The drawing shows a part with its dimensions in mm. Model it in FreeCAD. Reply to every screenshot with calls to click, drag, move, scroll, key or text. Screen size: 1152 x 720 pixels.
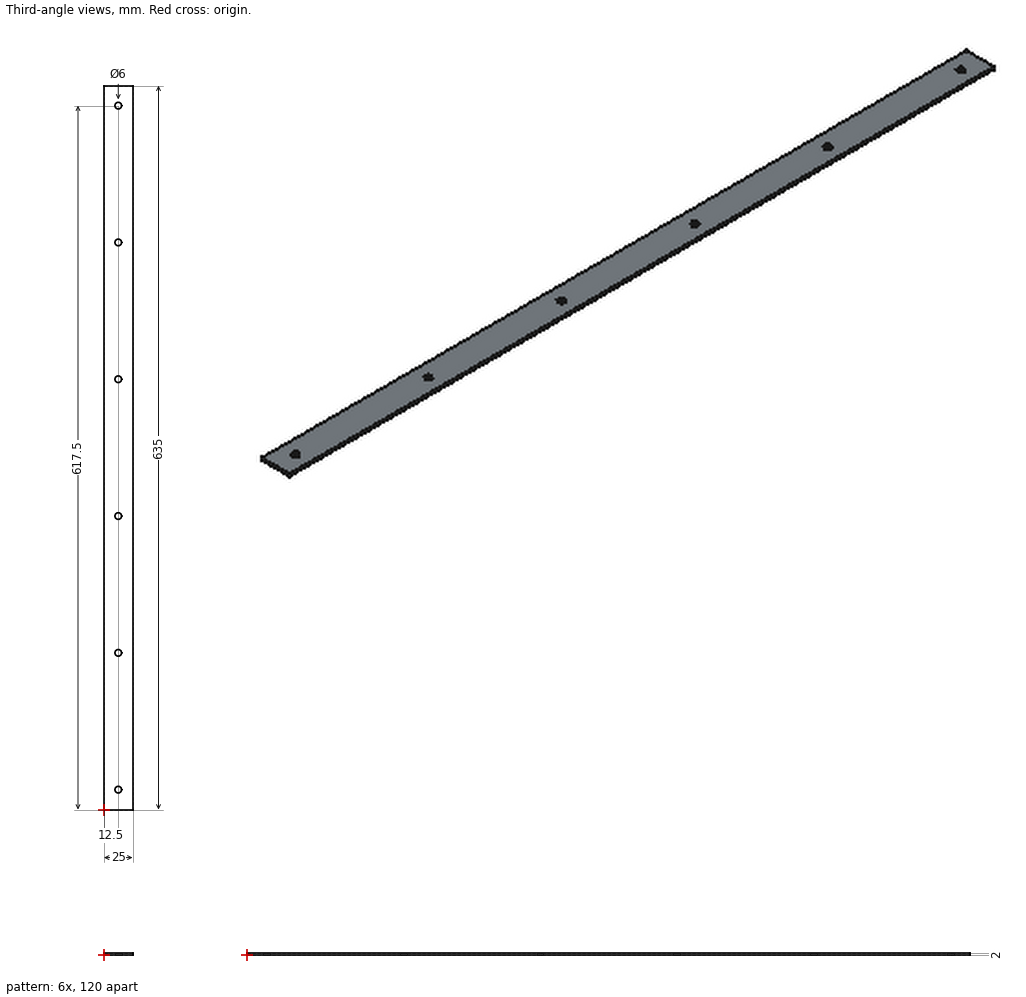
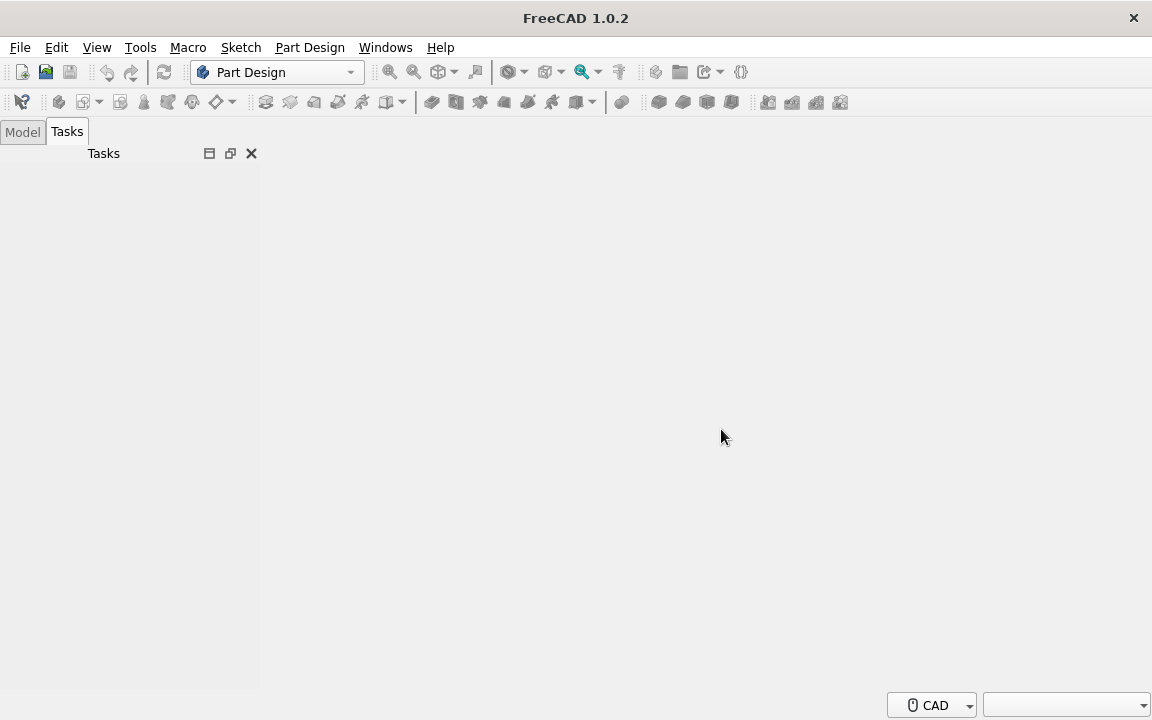
key(ctrl+n)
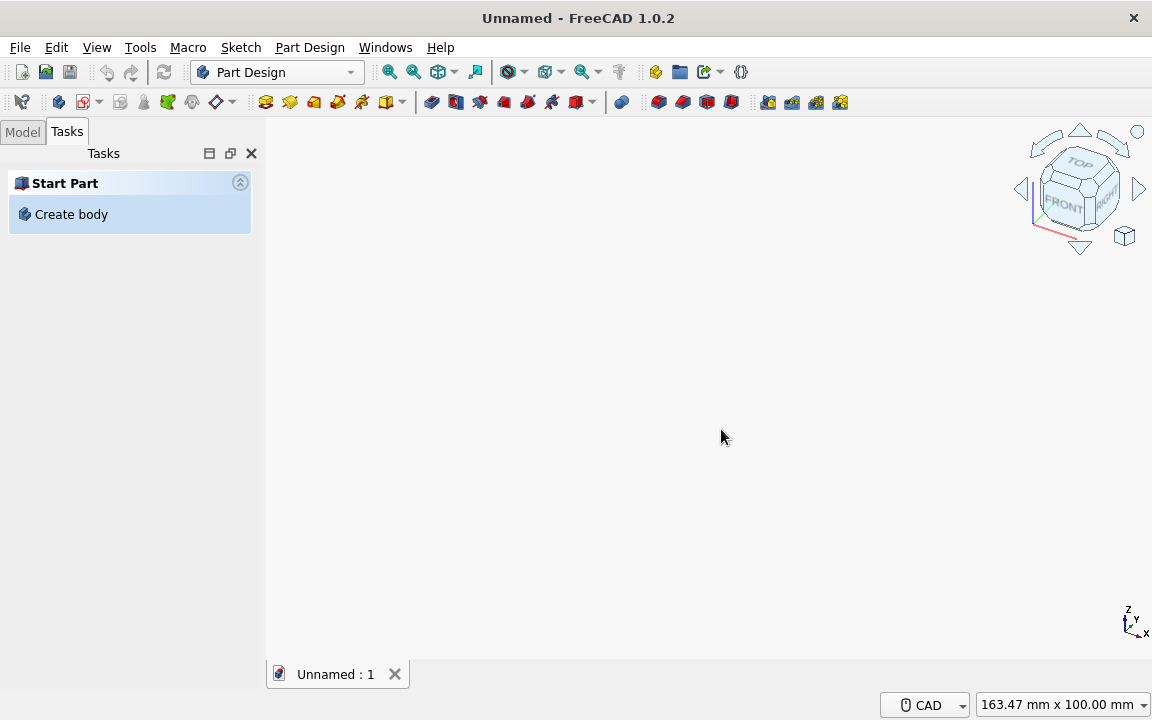
click(84, 102)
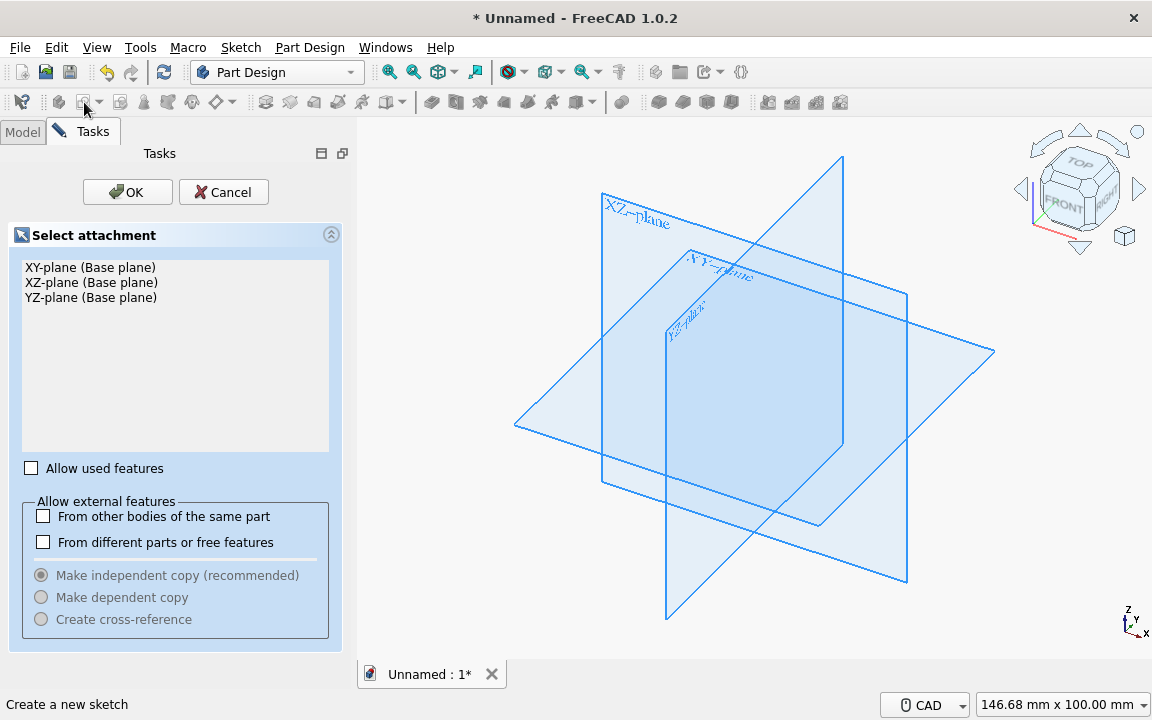
click(82, 268)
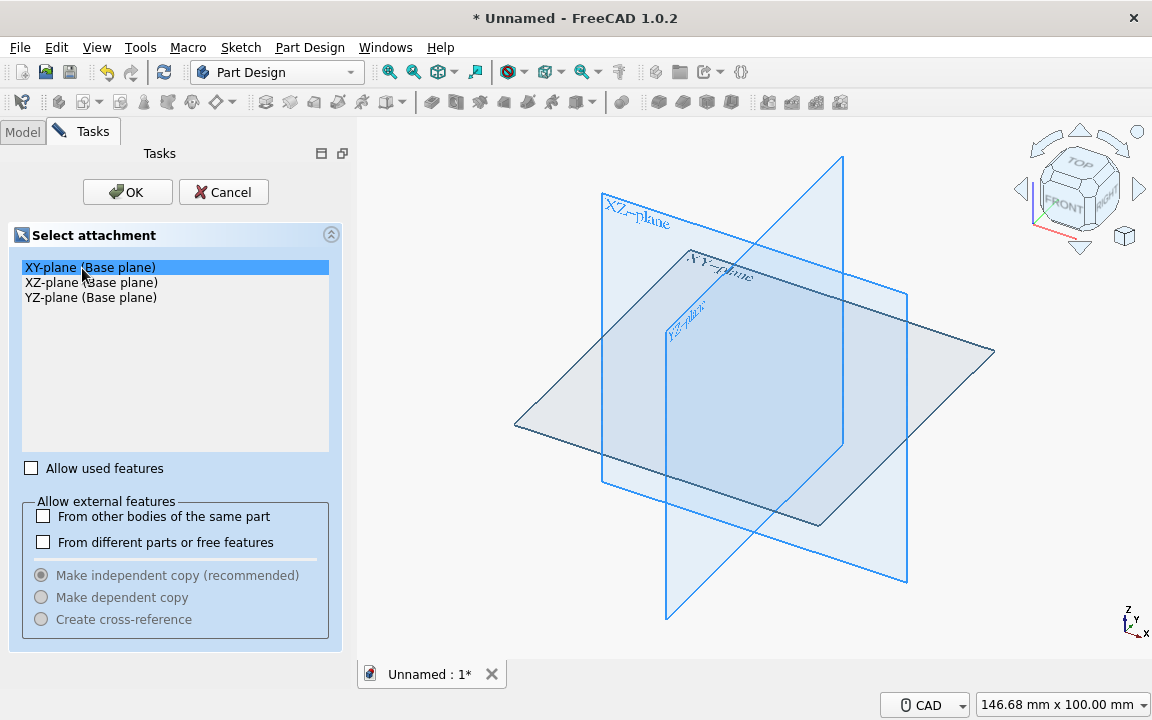
click(128, 192)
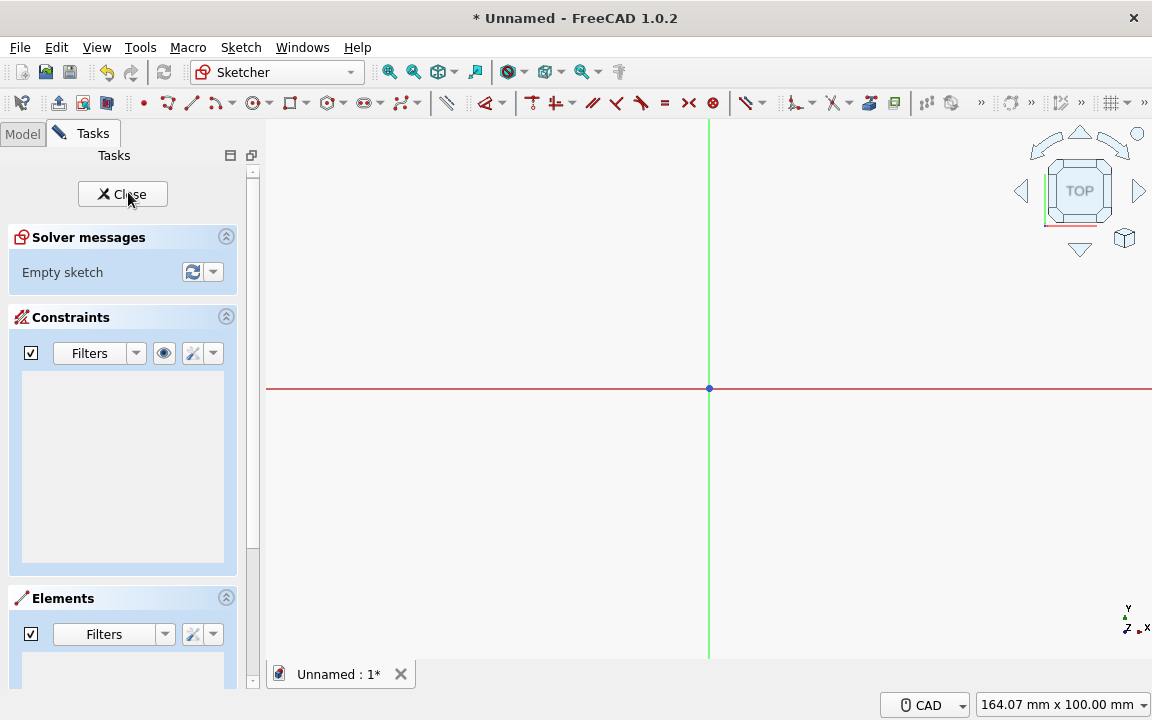
scroll(627, 560, down, 12)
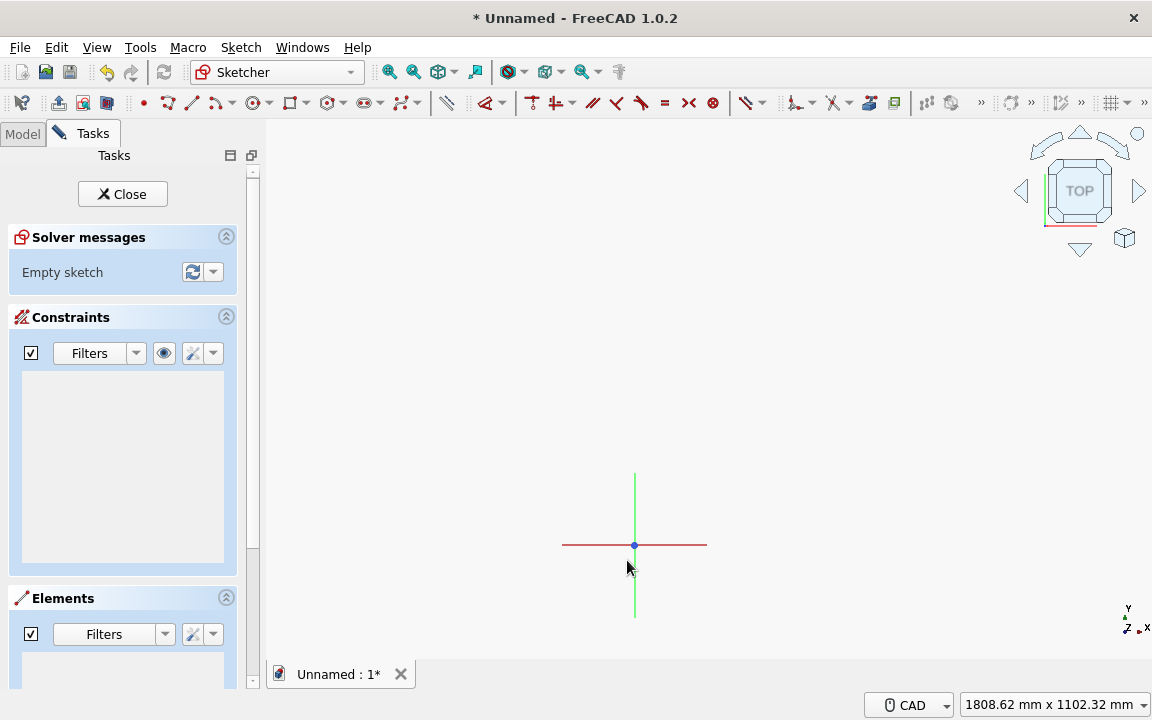
click(290, 104)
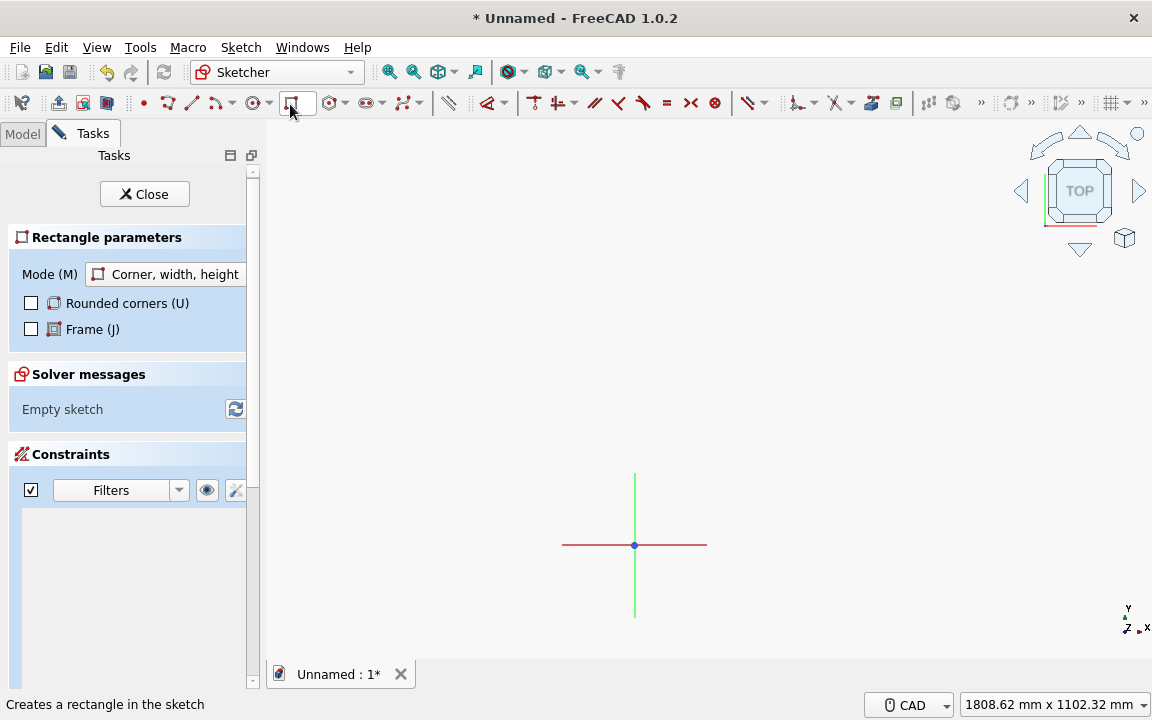
scroll(635, 545, up, 2)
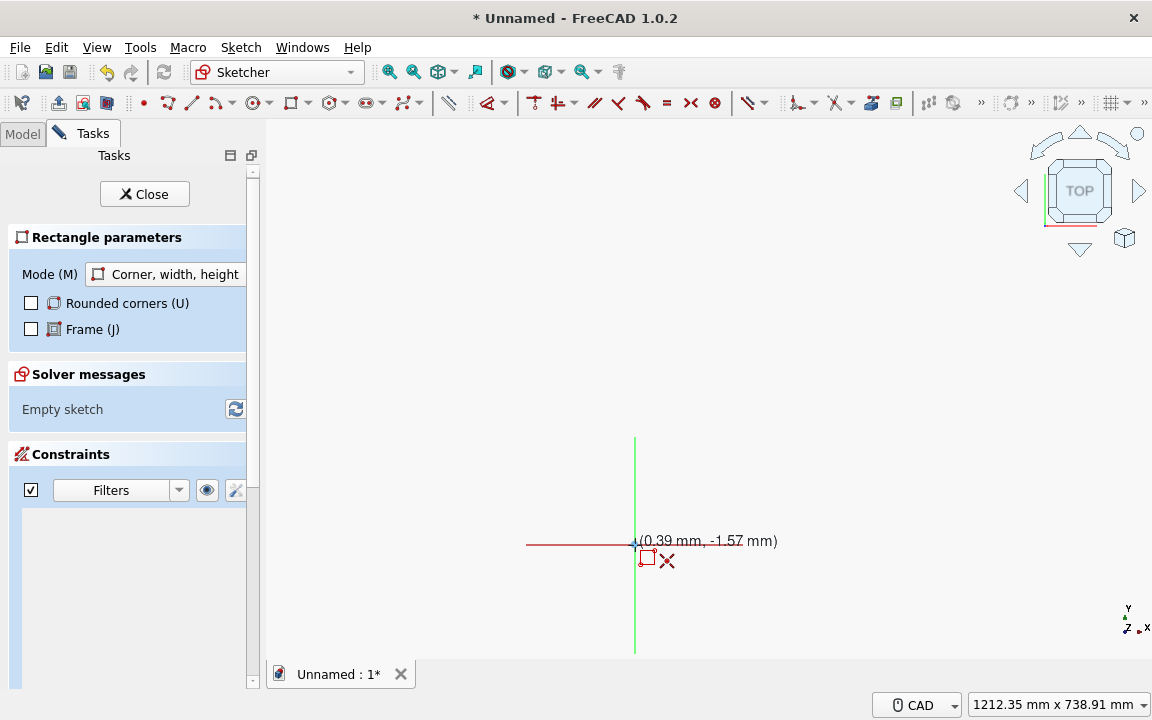
click(635, 545)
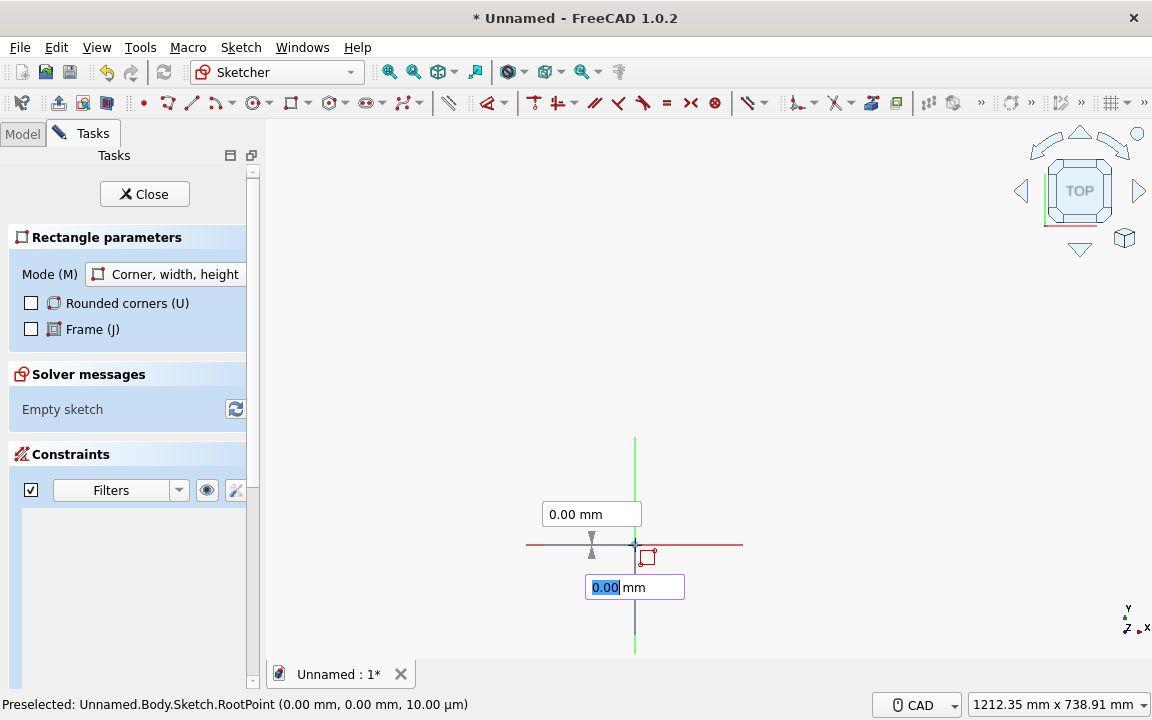
scroll(634, 544, down, 2)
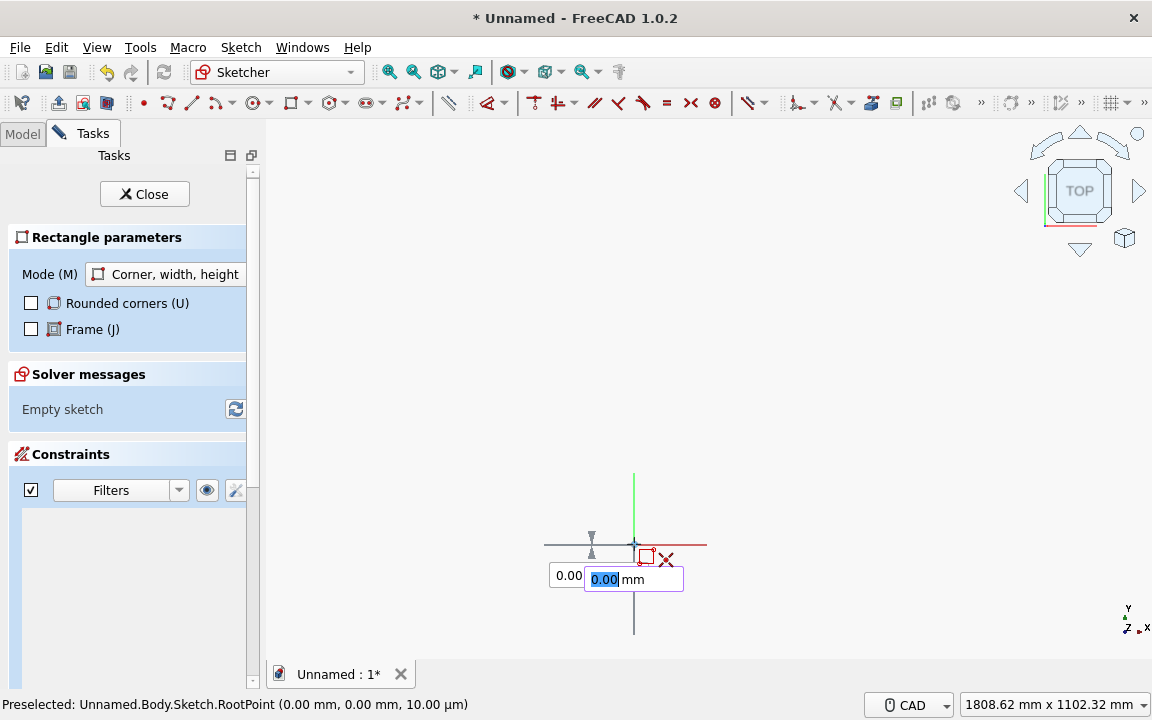
scroll(647, 234, up, 2)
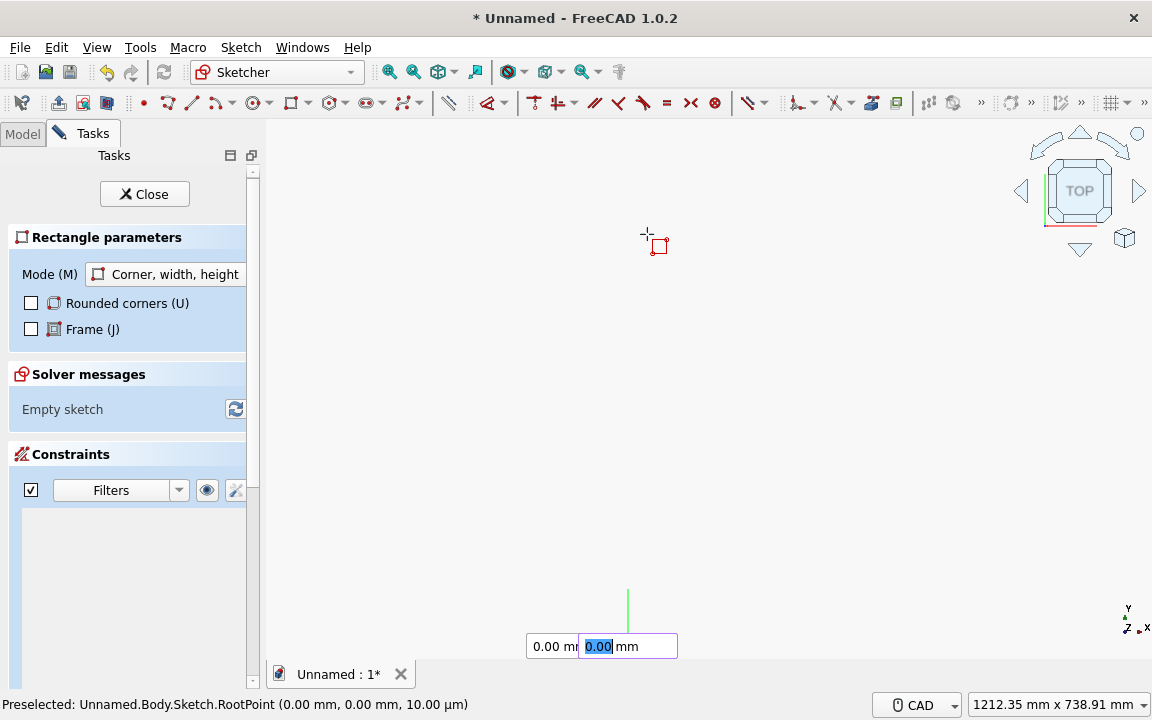
click(646, 234)
key(Escape)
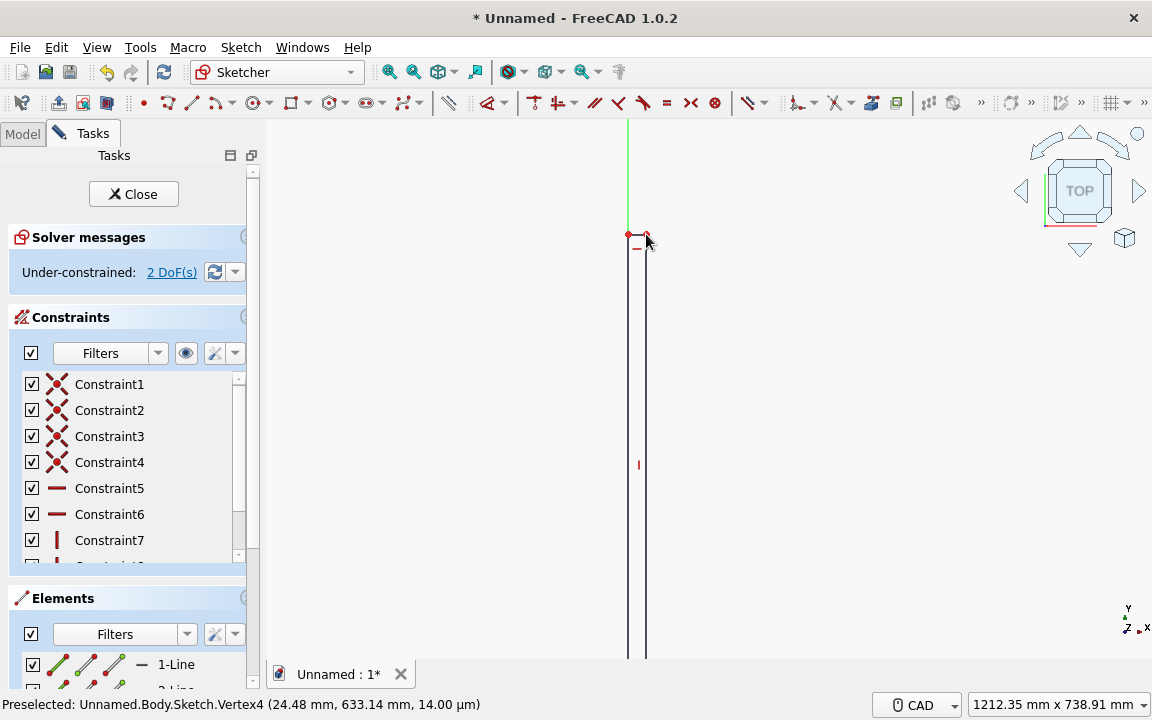
scroll(647, 233, down, 2)